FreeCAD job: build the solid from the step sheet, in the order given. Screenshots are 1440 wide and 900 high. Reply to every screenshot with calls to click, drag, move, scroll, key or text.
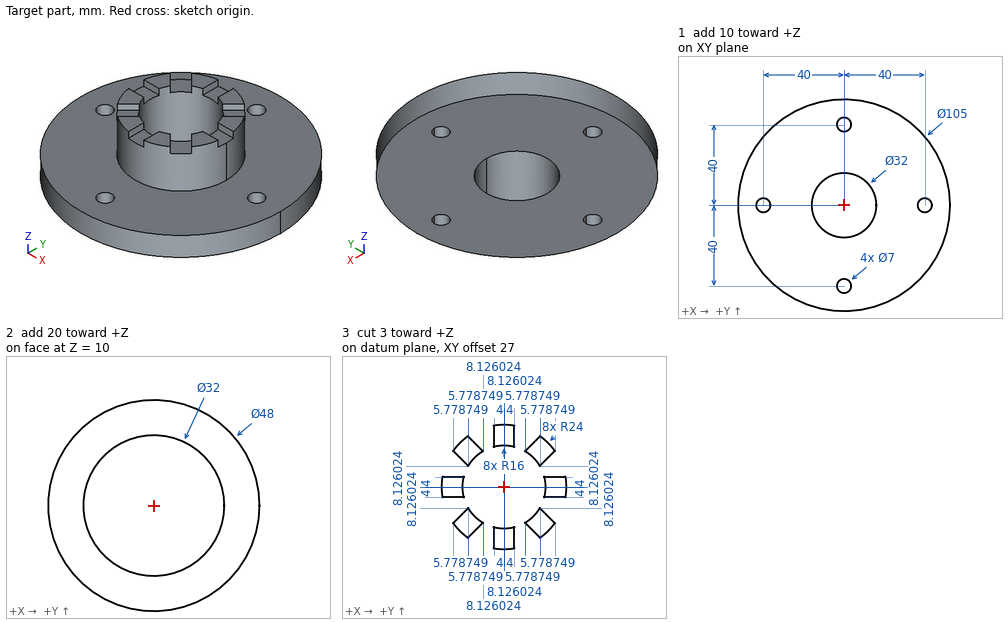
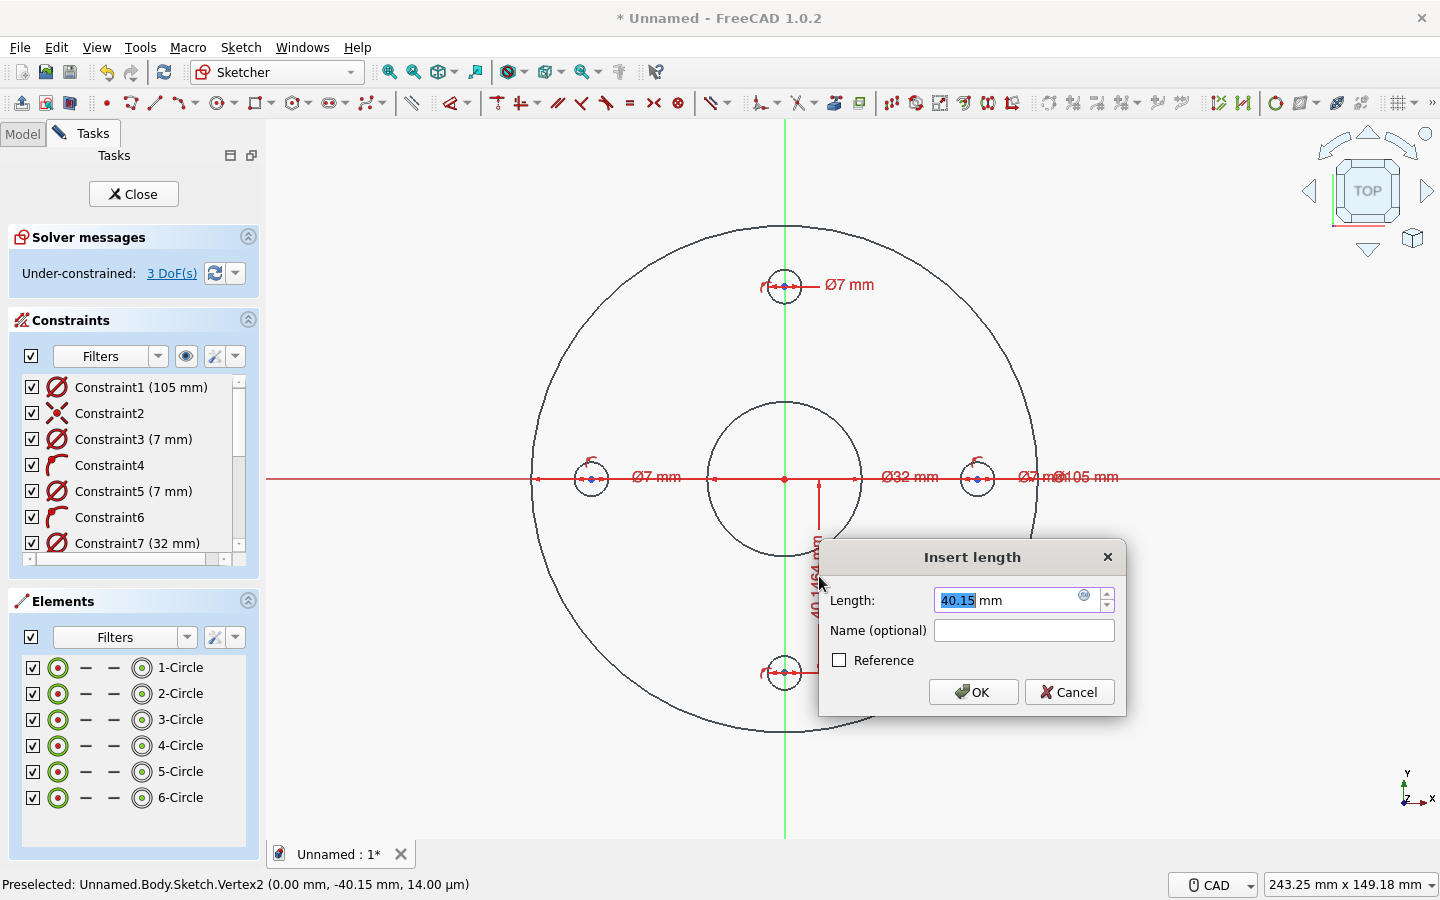
text(40)
key(Return)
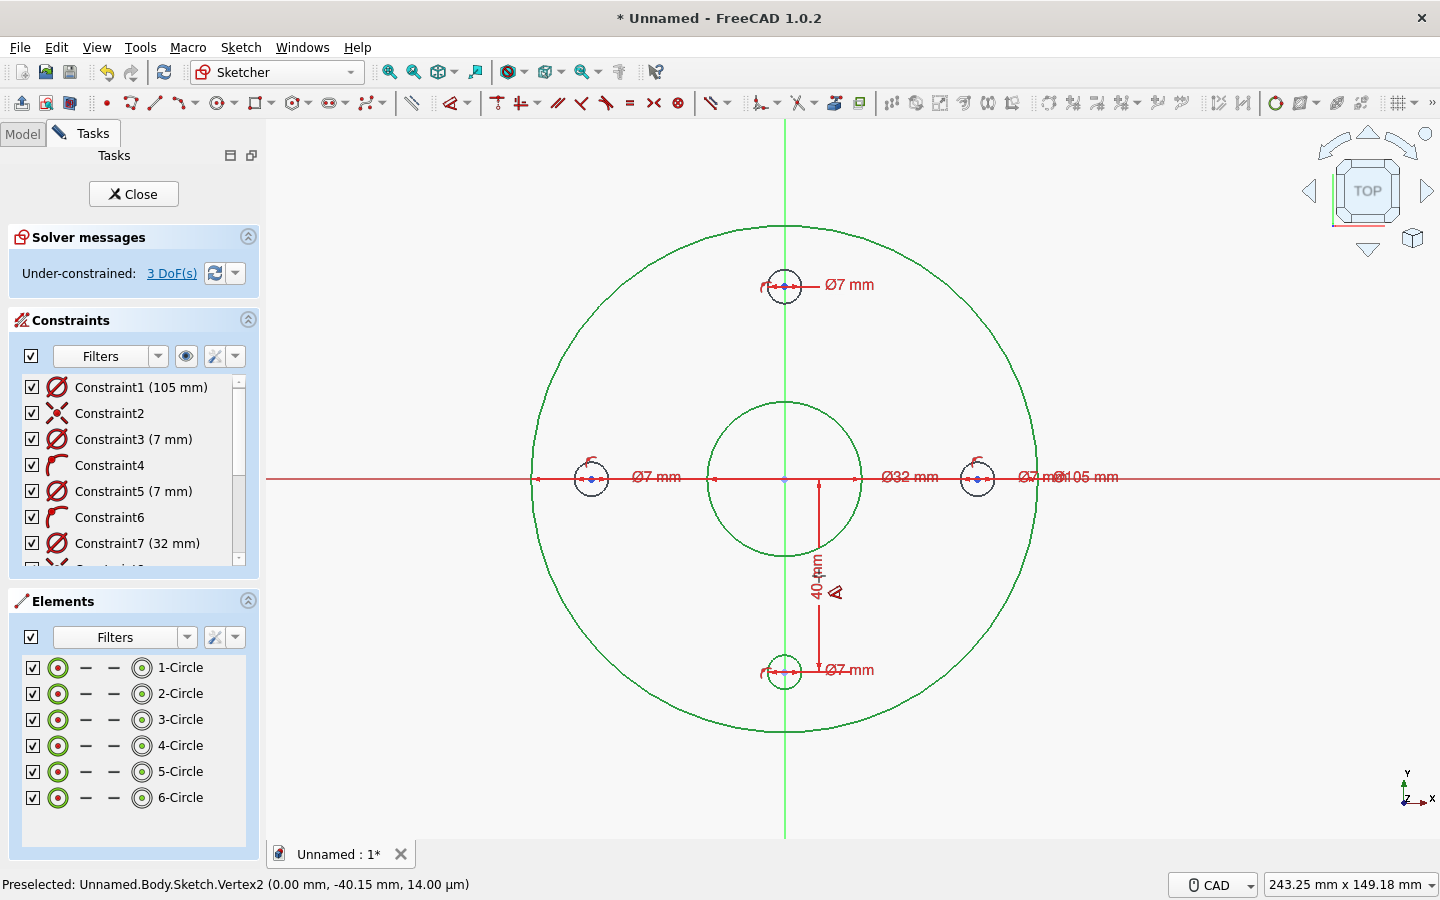
click(591, 479)
click(688, 513)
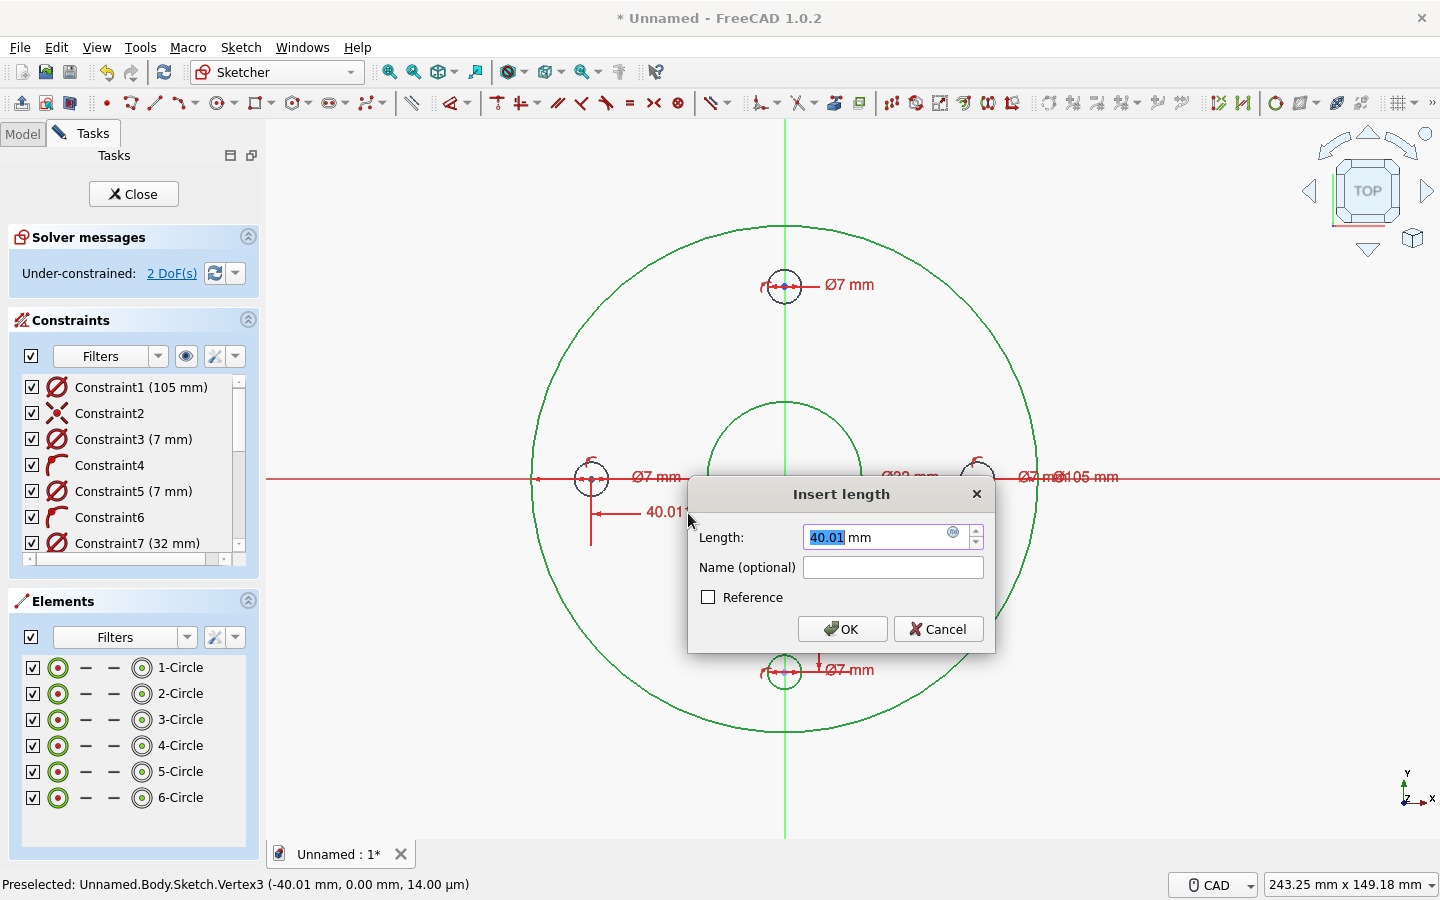
text(40)
key(Return)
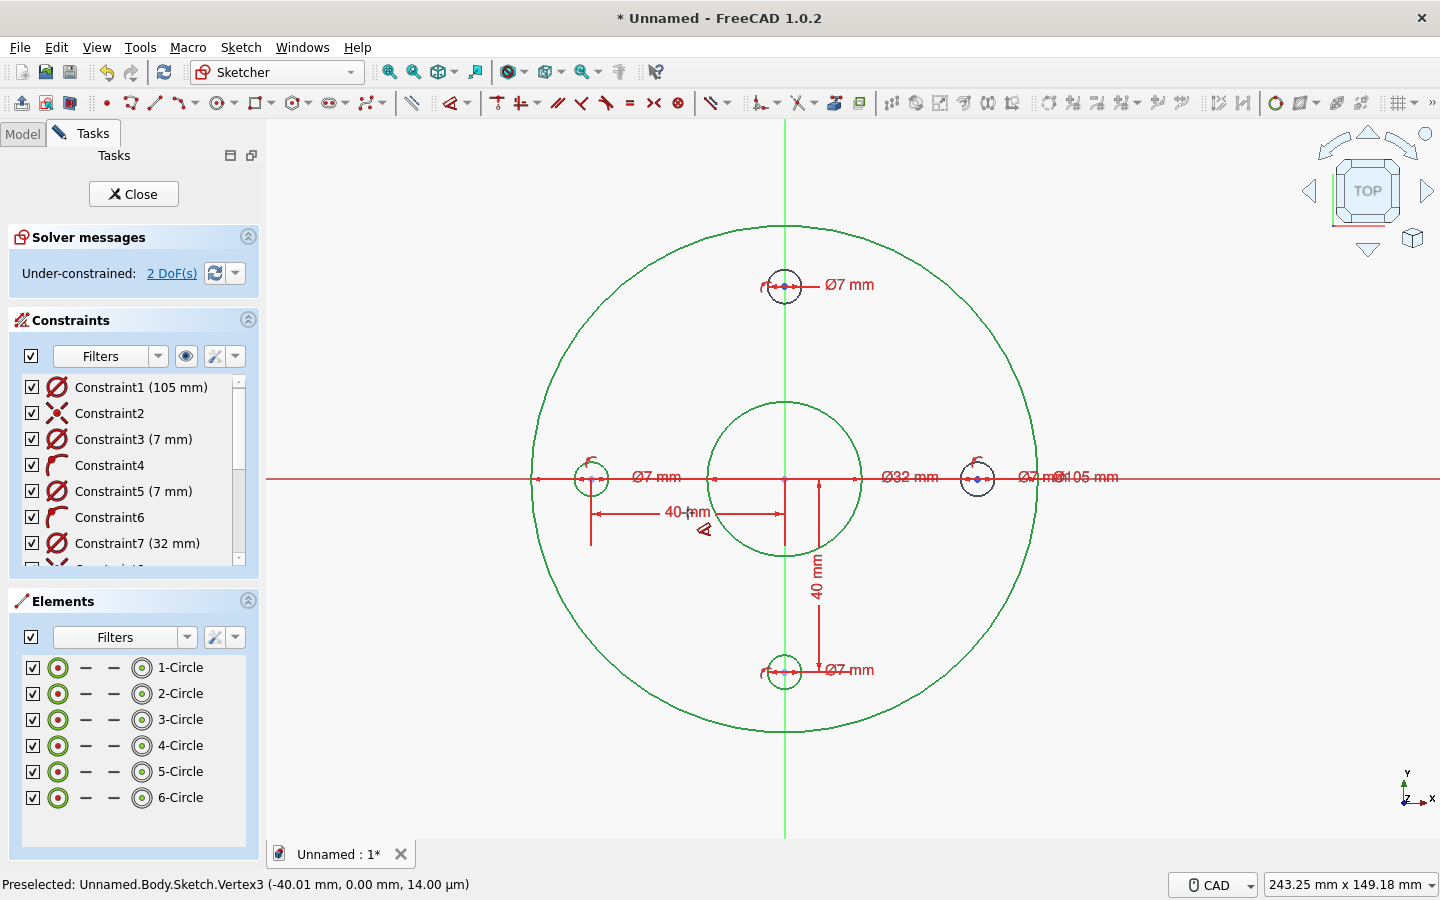
click(978, 479)
click(881, 513)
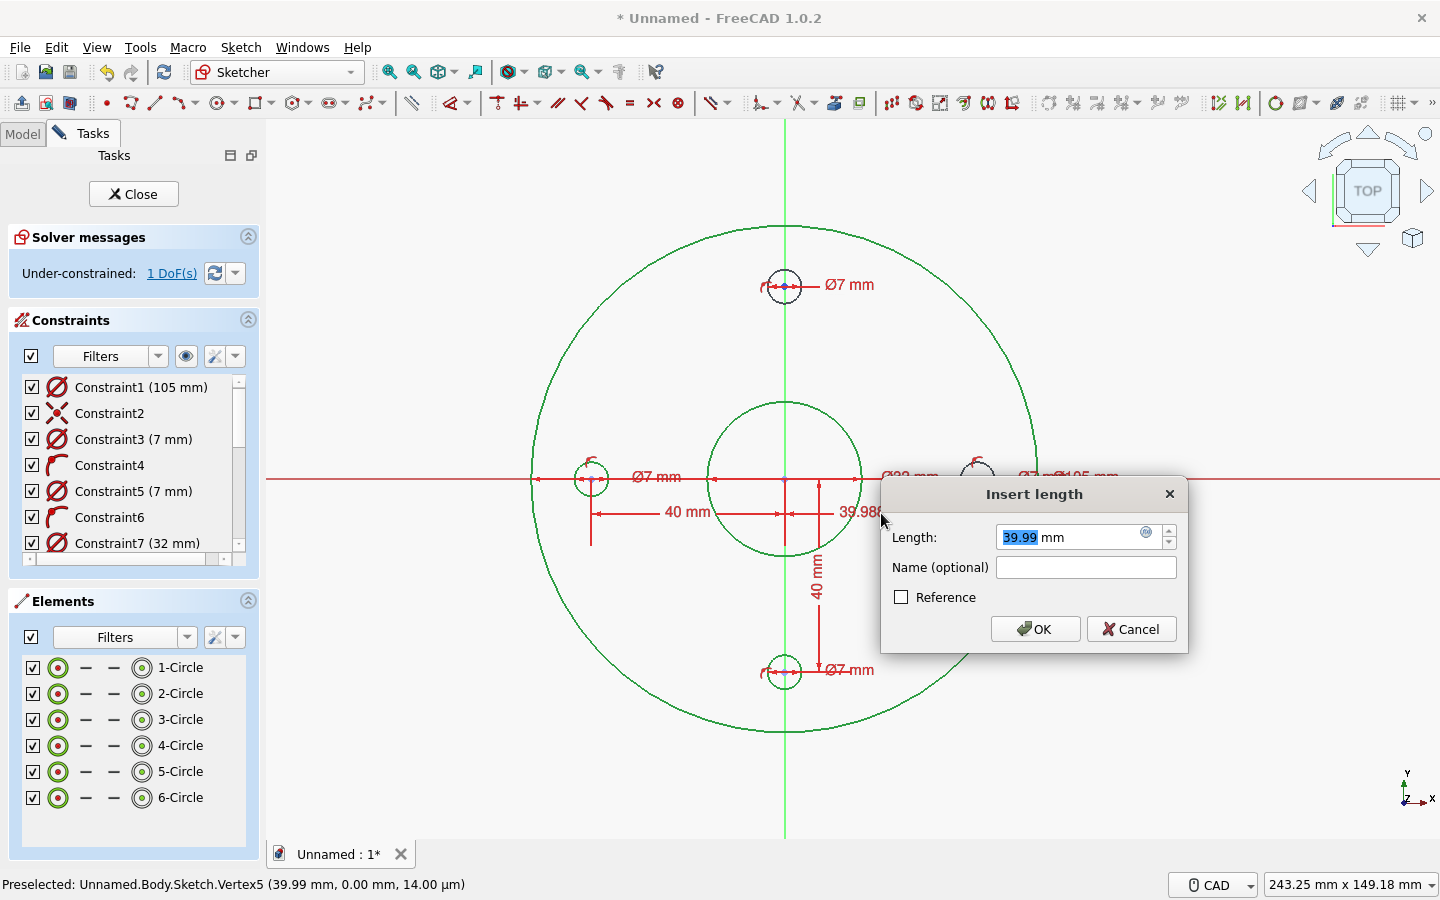
text(40)
key(Return)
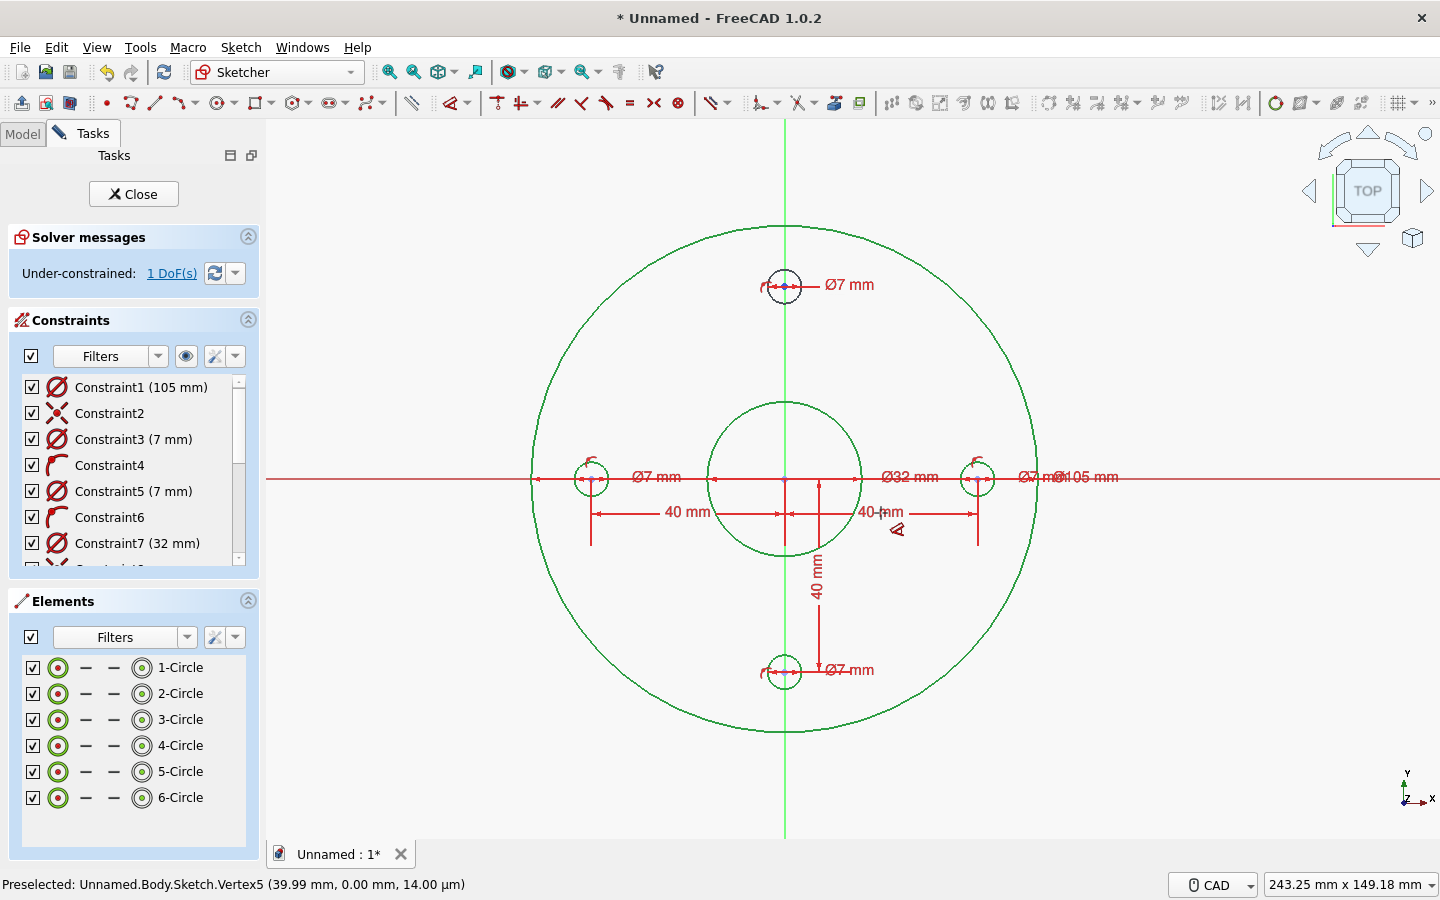
click(785, 287)
click(819, 383)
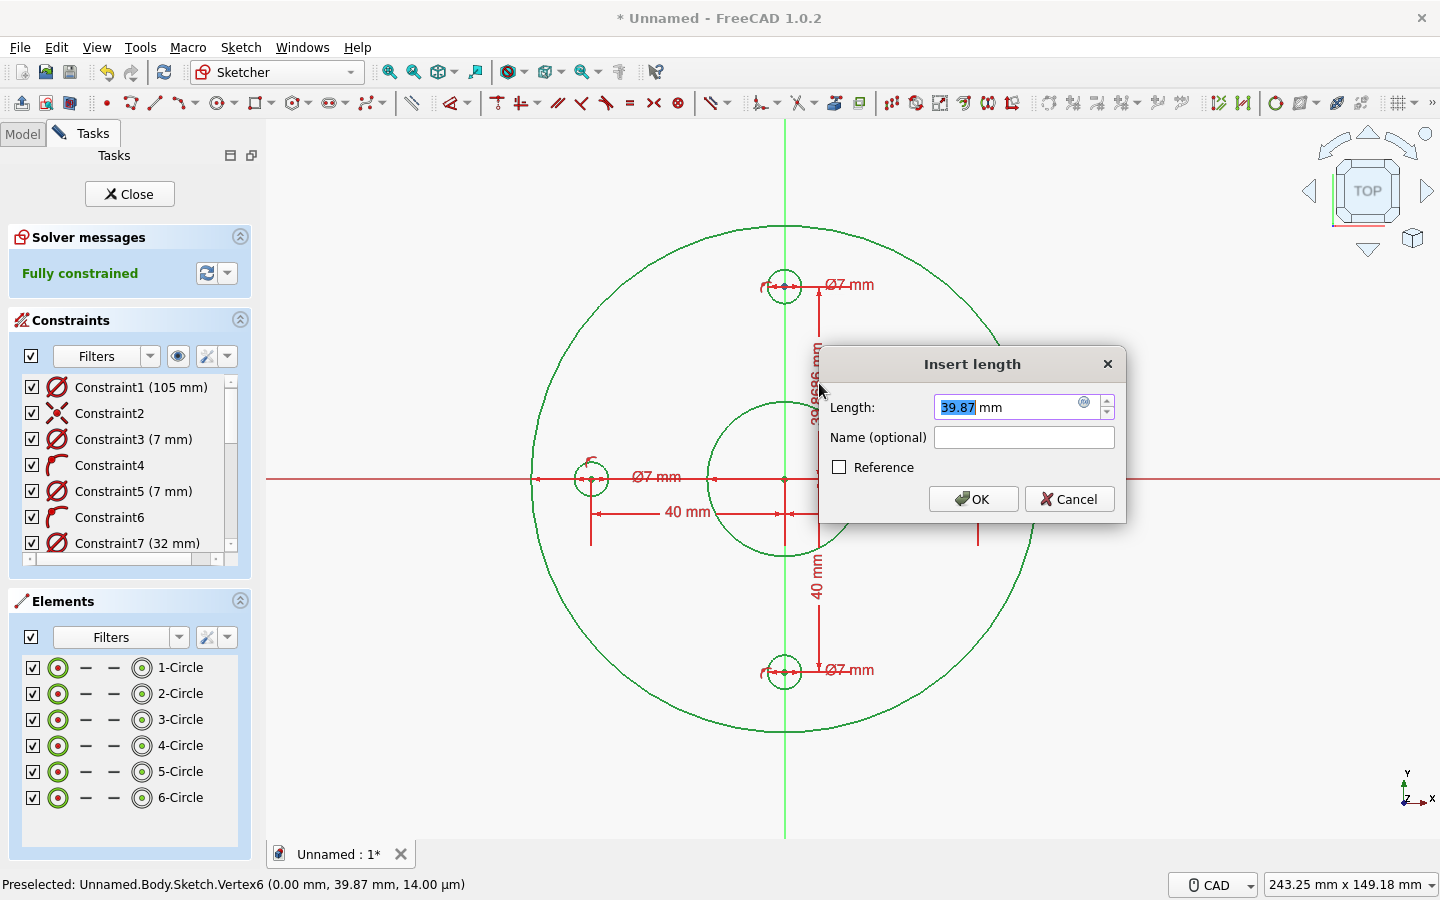
text(40)
key(Return)
key(Escape)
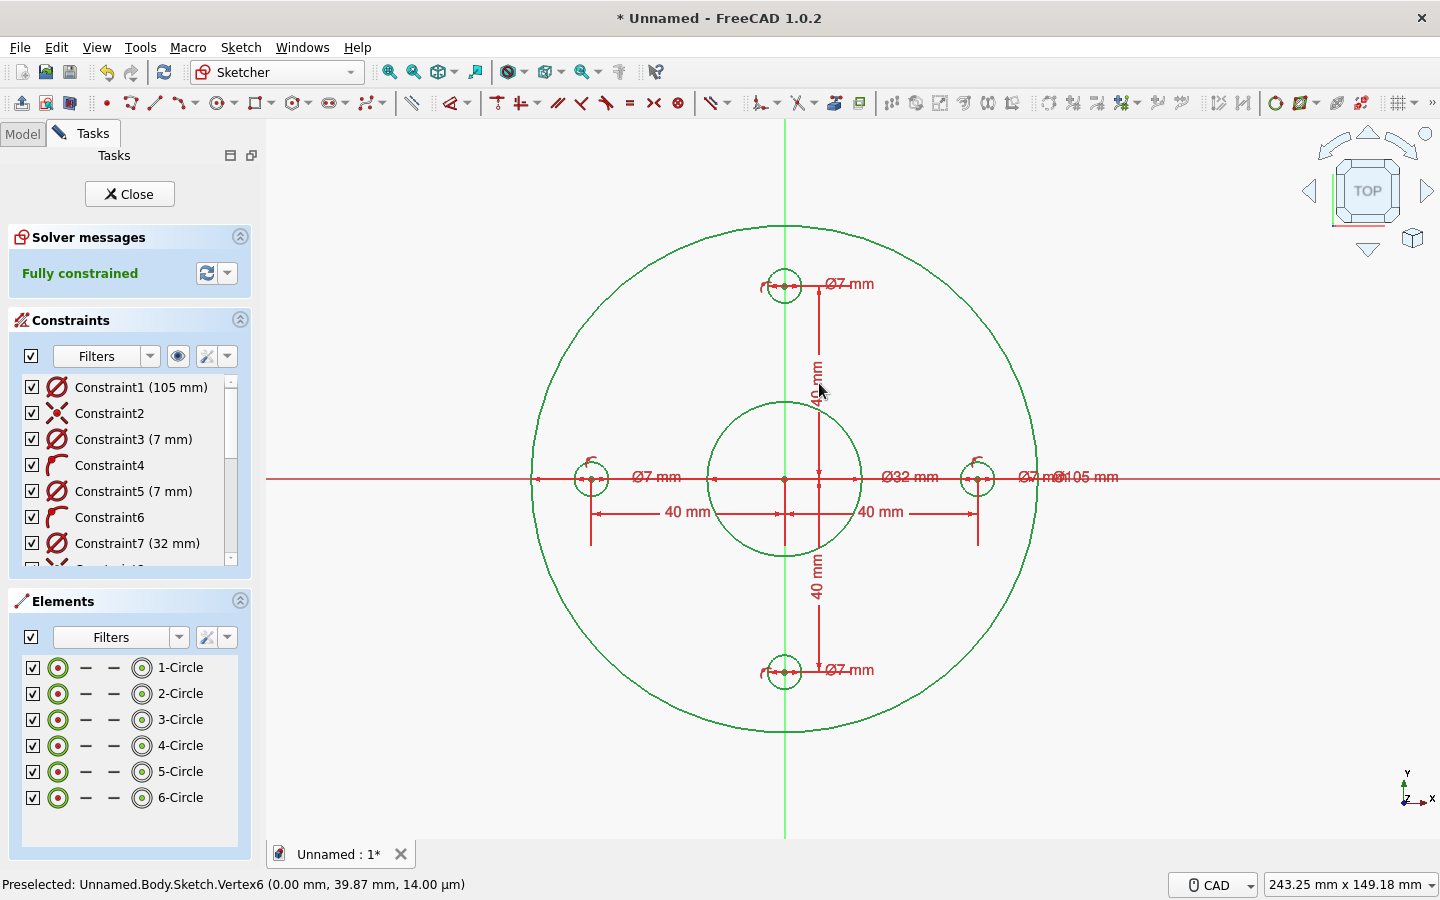
click(130, 194)